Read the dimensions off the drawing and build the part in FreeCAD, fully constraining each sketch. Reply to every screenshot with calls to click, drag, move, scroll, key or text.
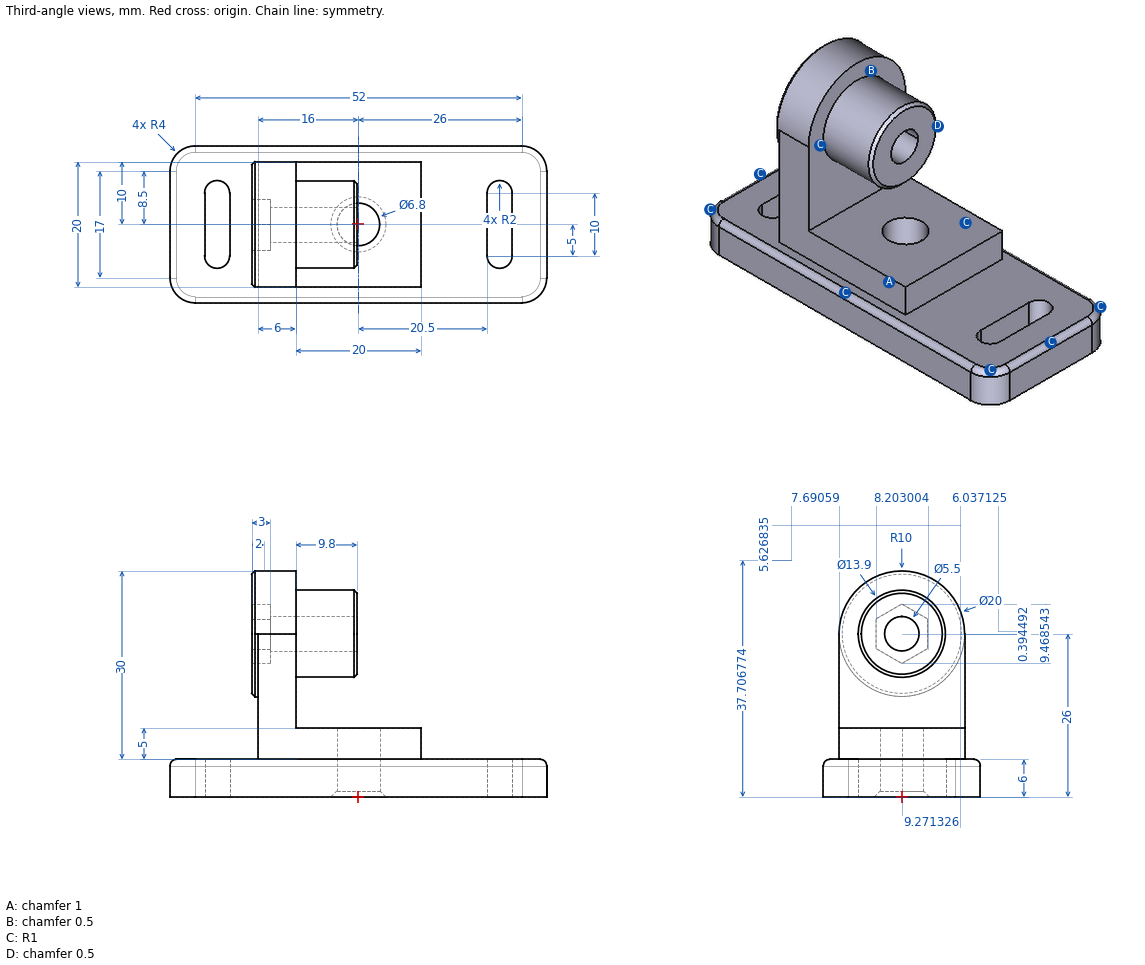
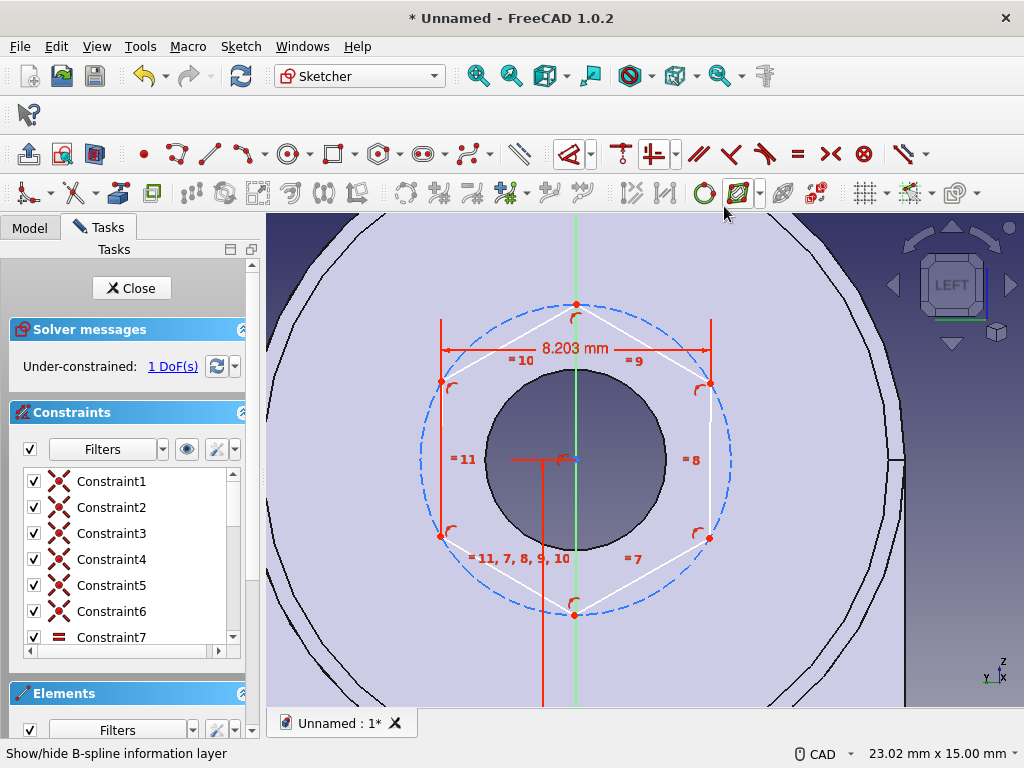
click(575, 615)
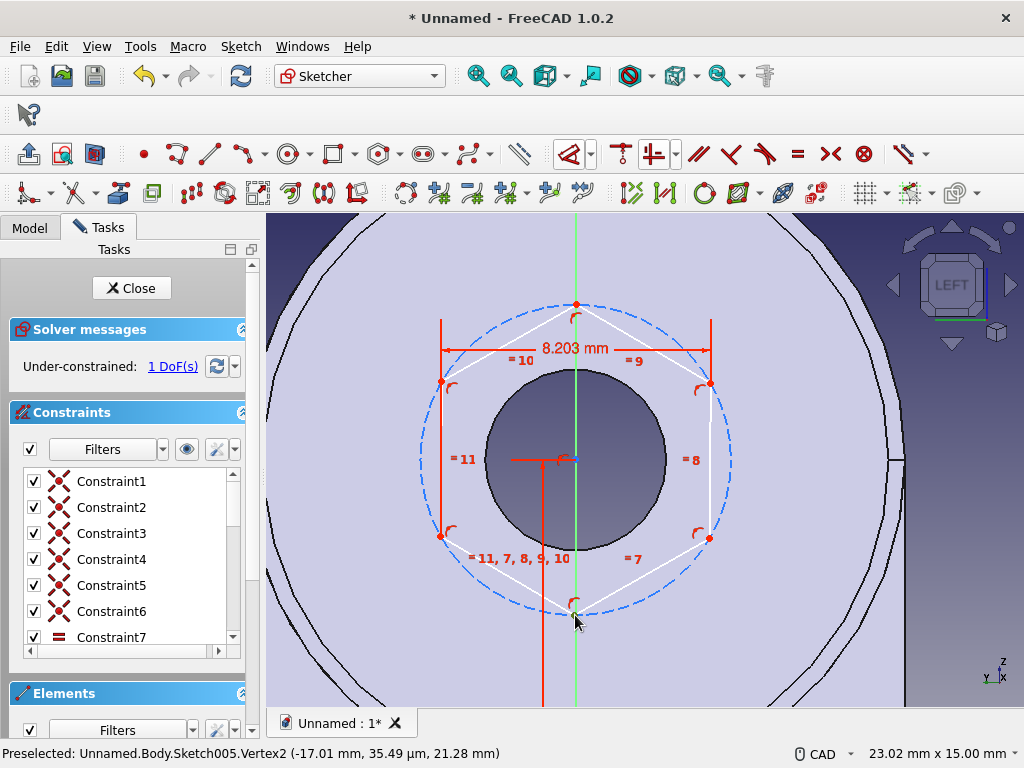
click(577, 305)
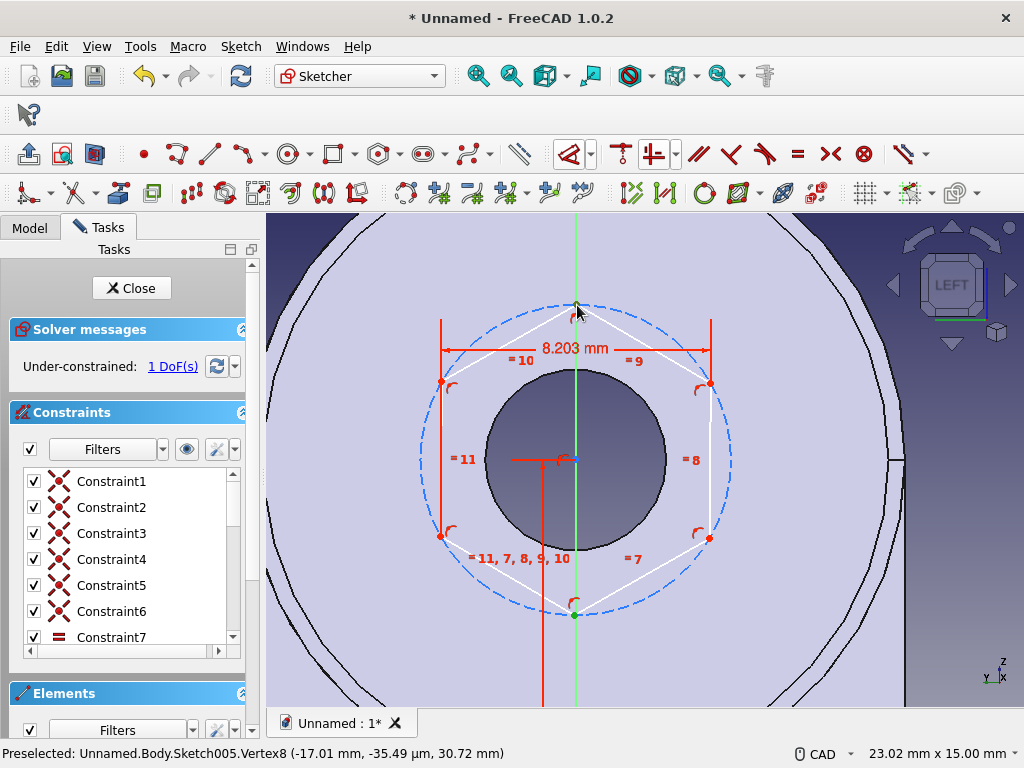
key(i)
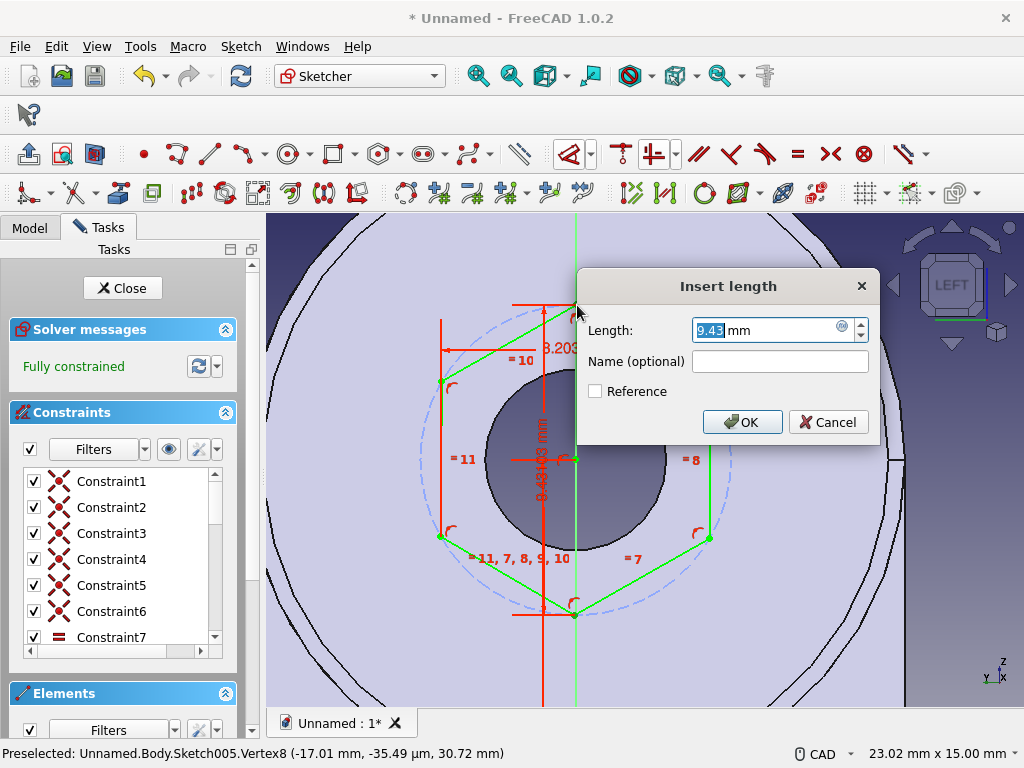
text(9.468543)
key(Return)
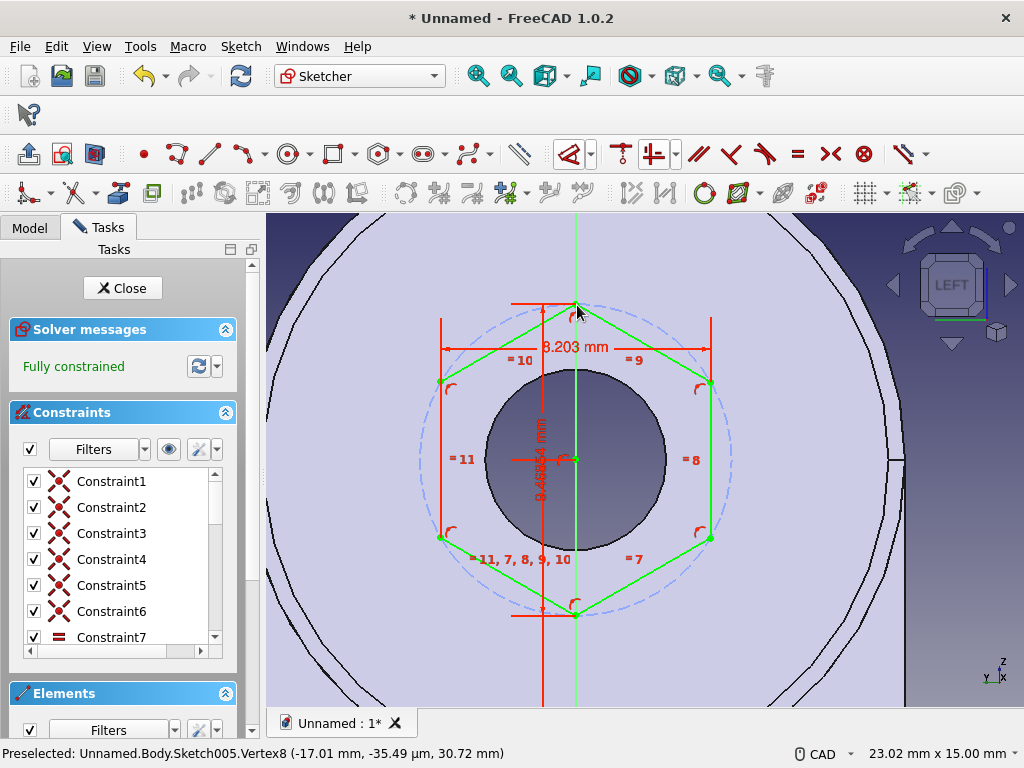
click(123, 288)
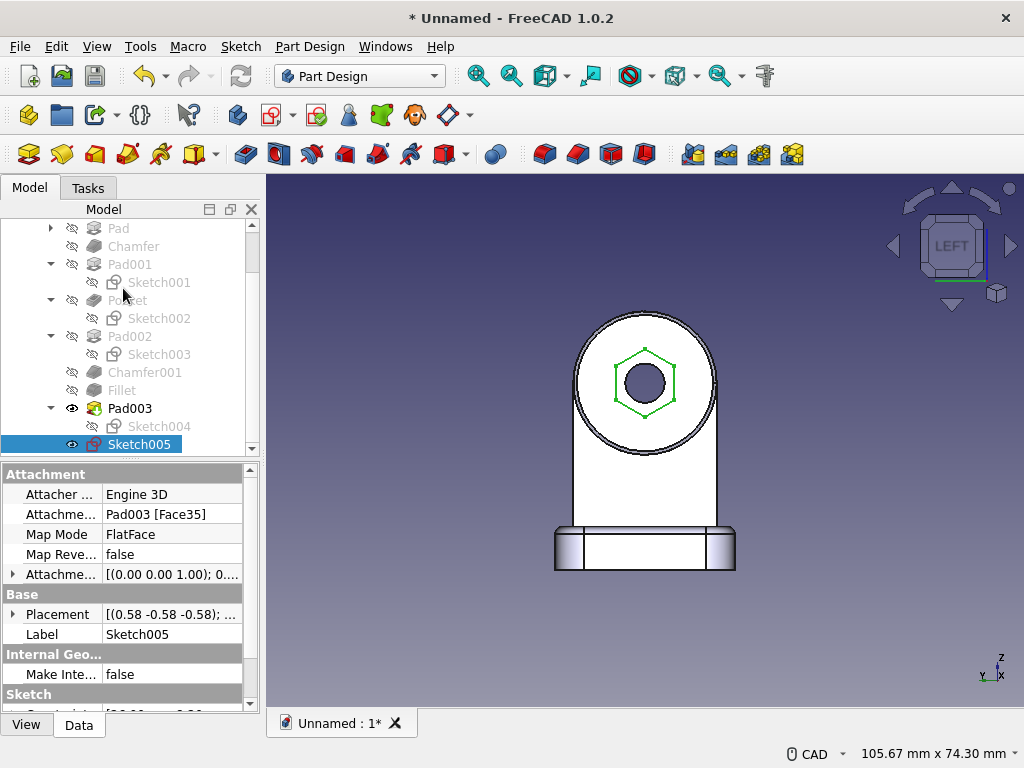
click(246, 154)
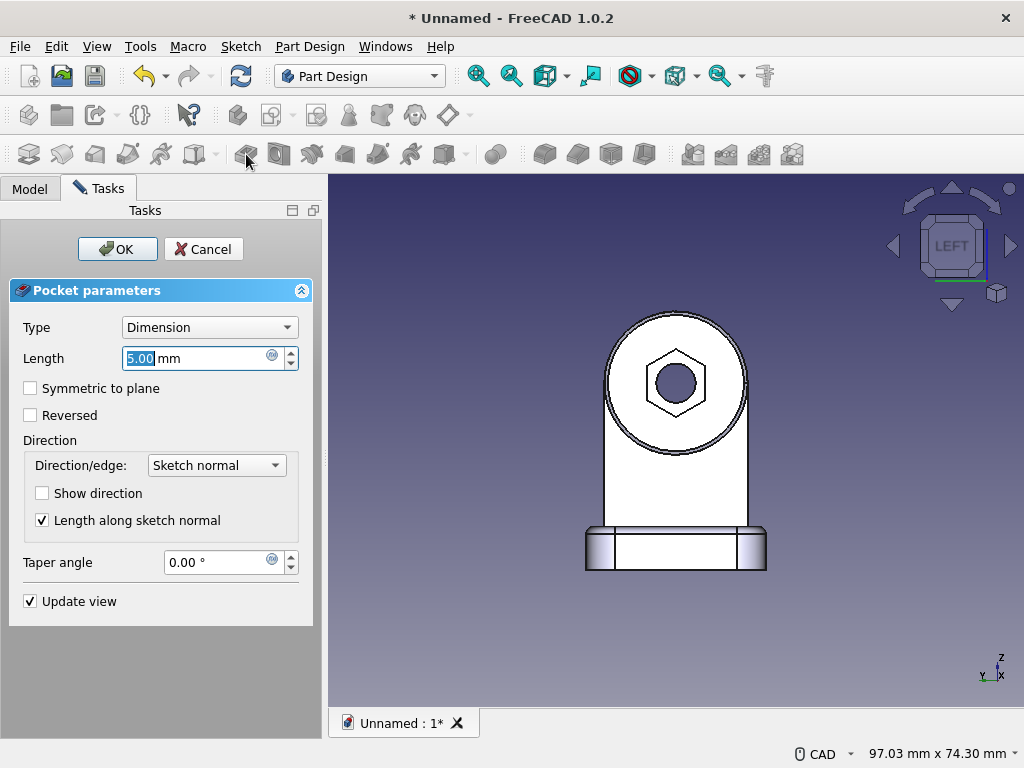
click(210, 328)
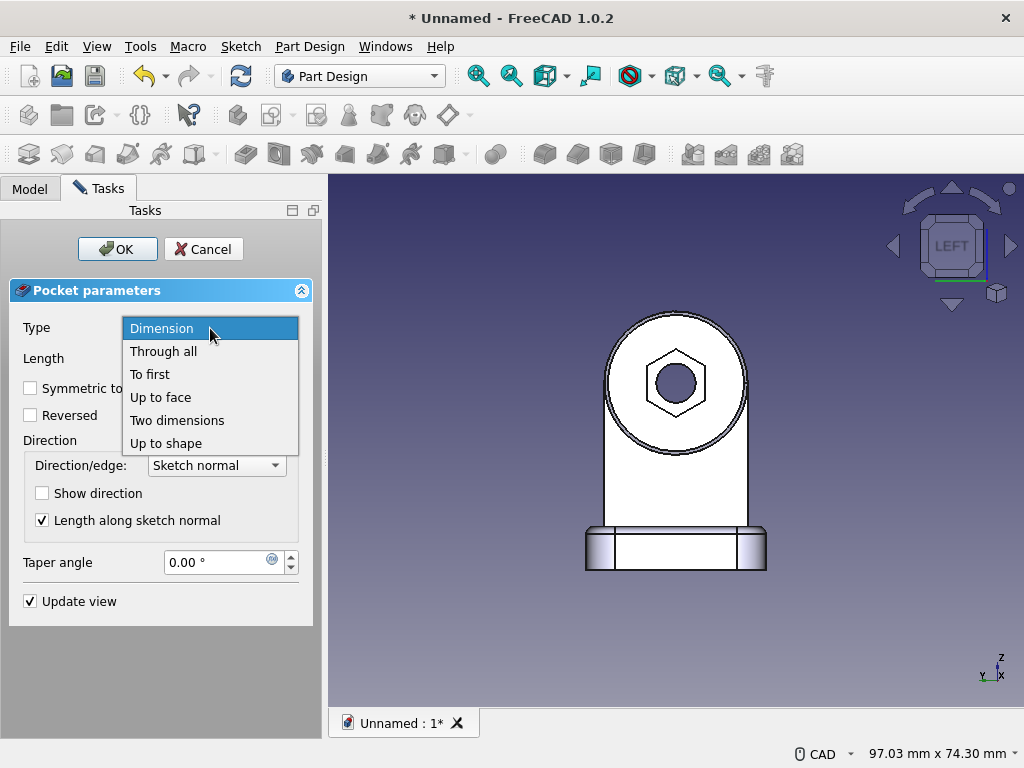
click(208, 420)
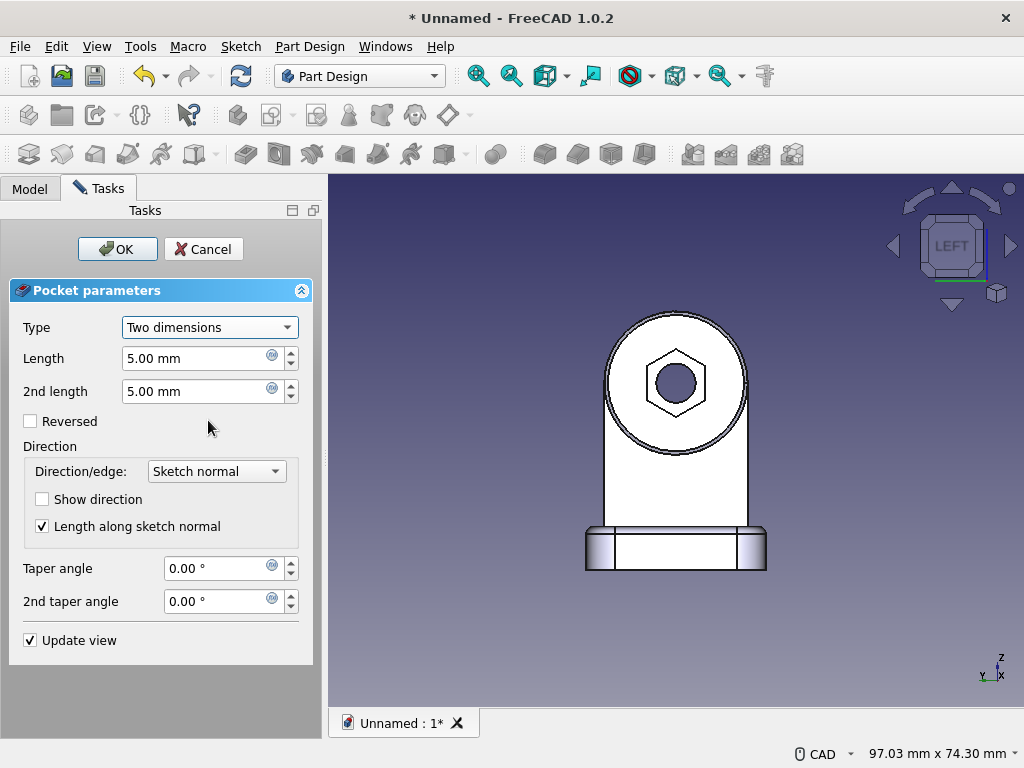
triple_click(204, 358)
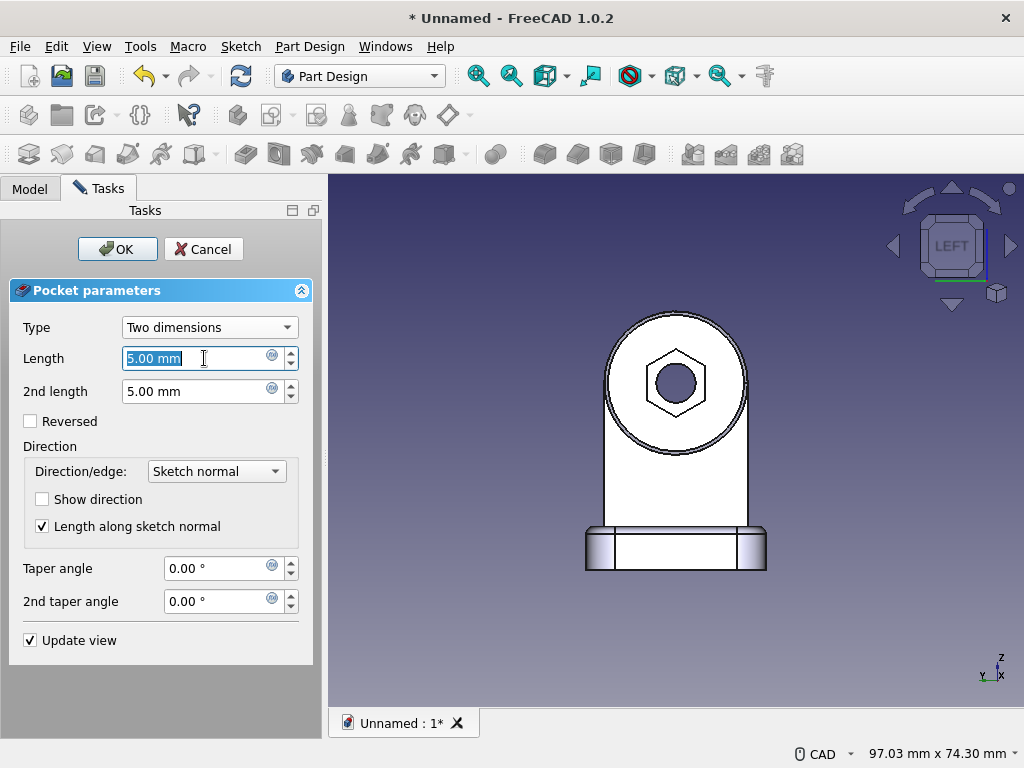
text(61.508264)
key(Tab)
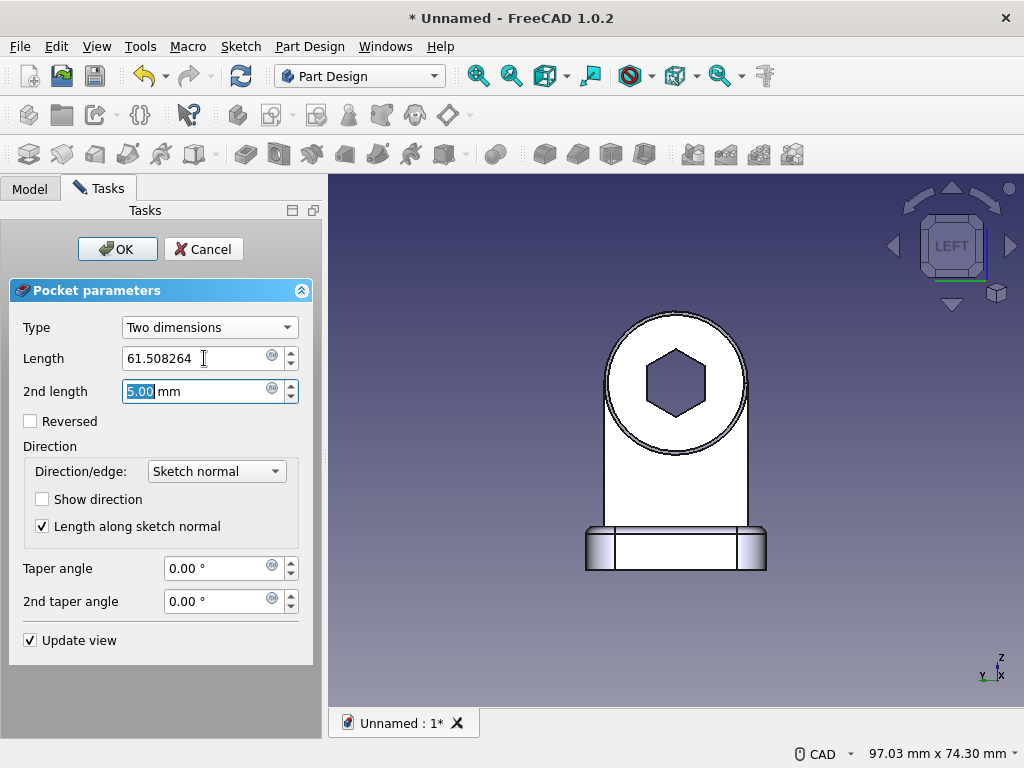
text(3)
key(Tab)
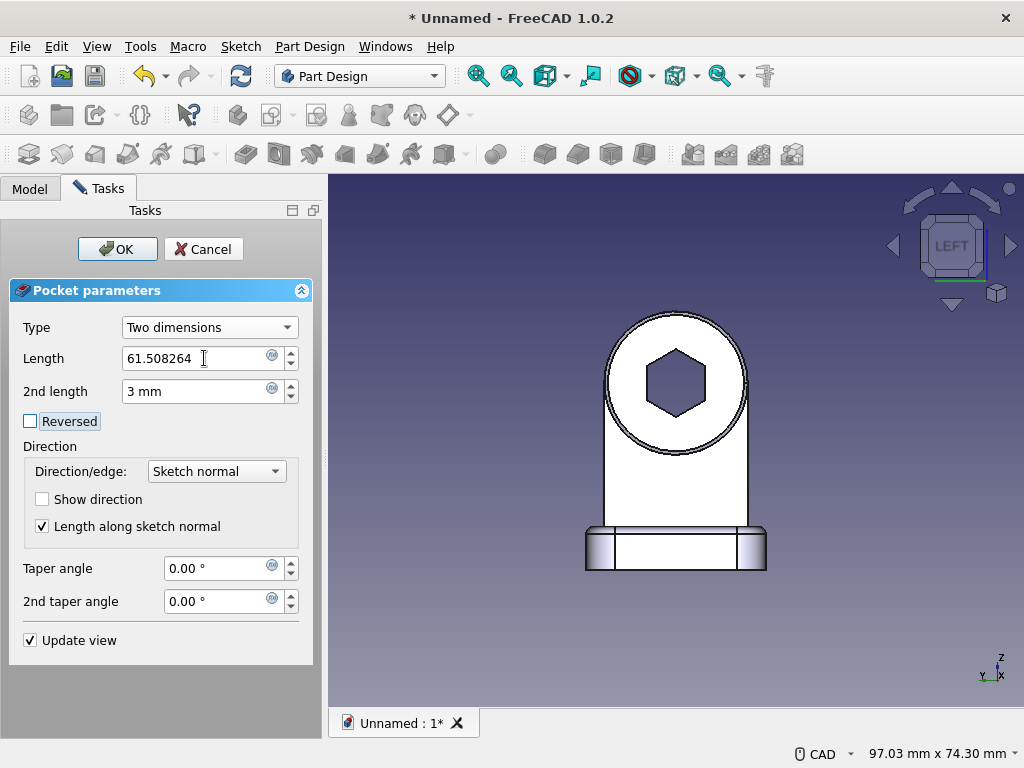
click(31, 421)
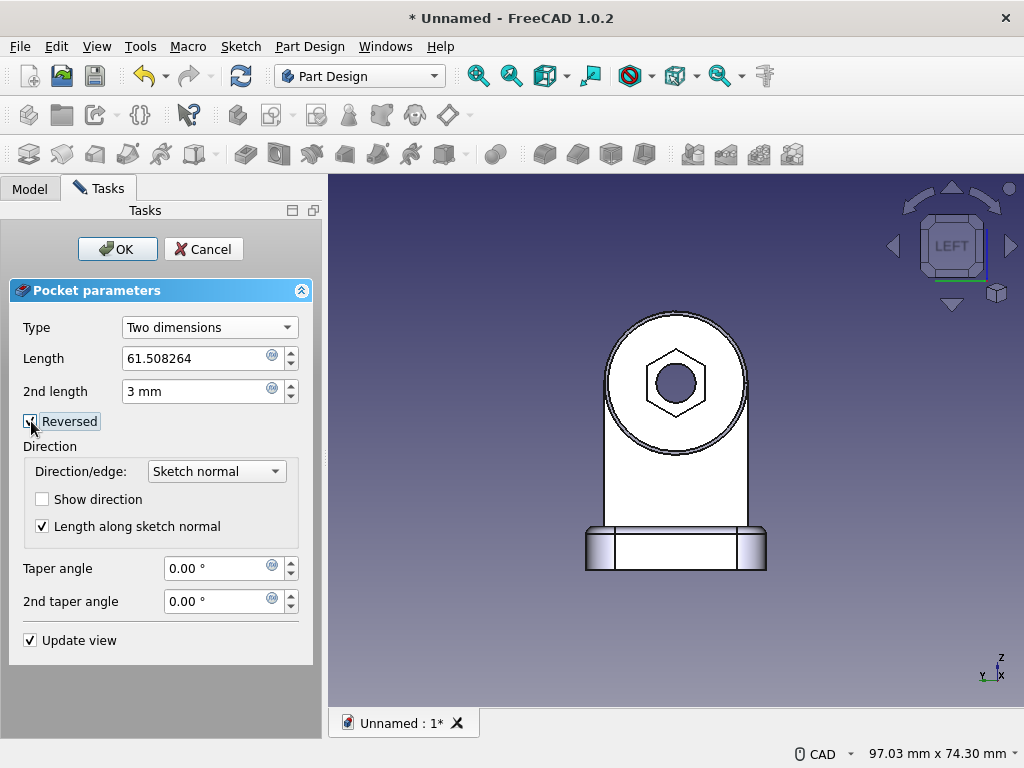
click(118, 249)